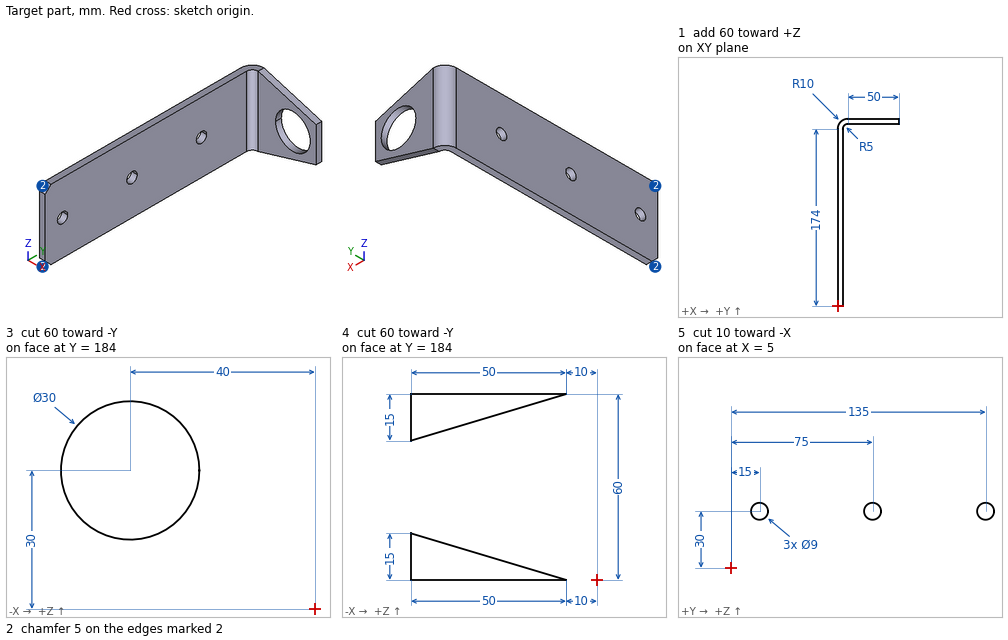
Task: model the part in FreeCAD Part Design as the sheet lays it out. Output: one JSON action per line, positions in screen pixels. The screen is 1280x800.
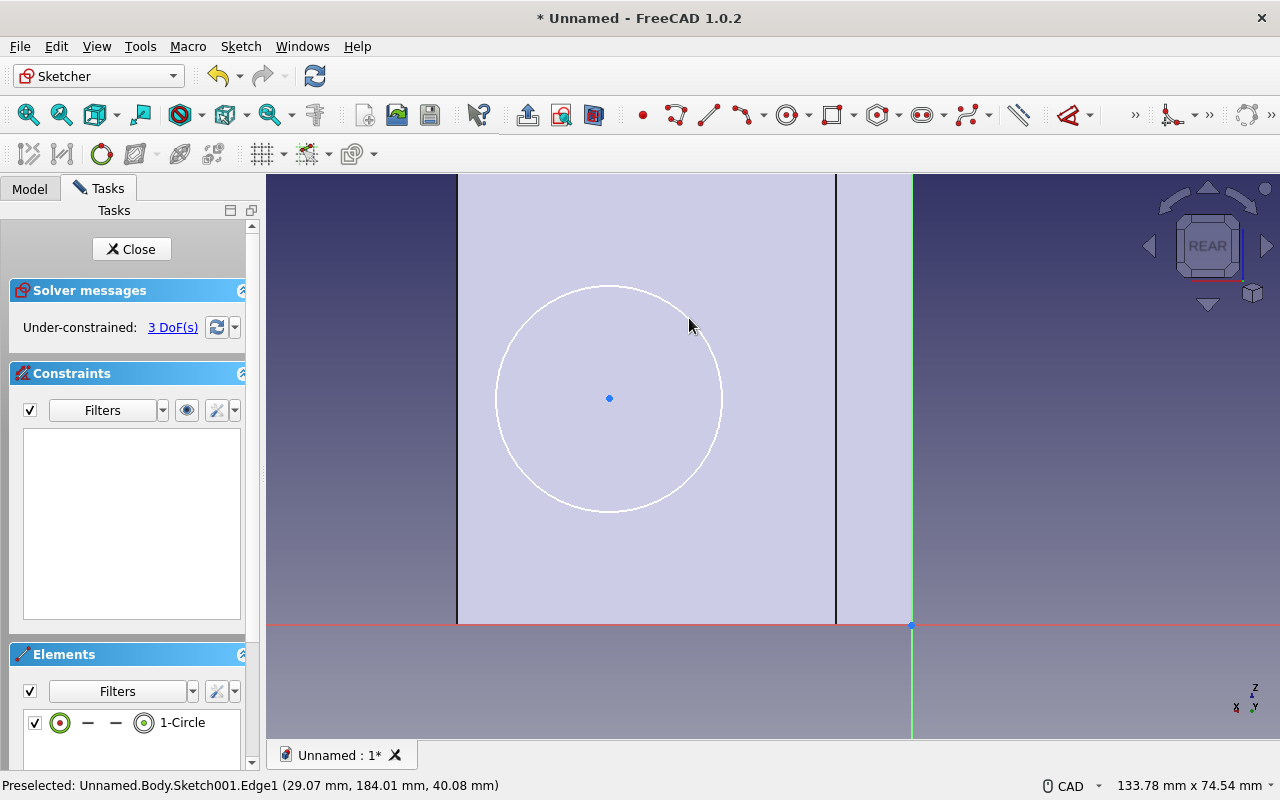
{"action": "key", "text": "d"}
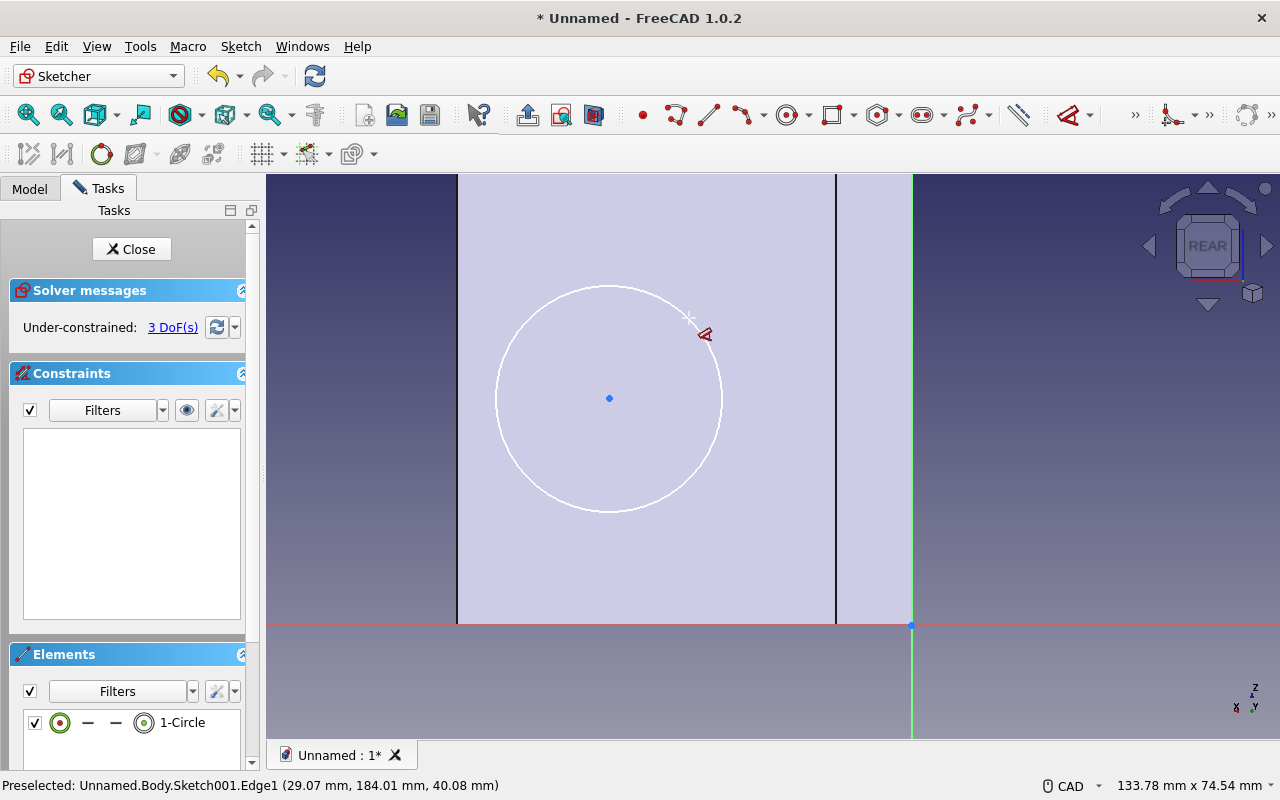
{"action": "left_click", "coordinate": [689, 319]}
{"action": "left_click", "coordinate": [712, 296]}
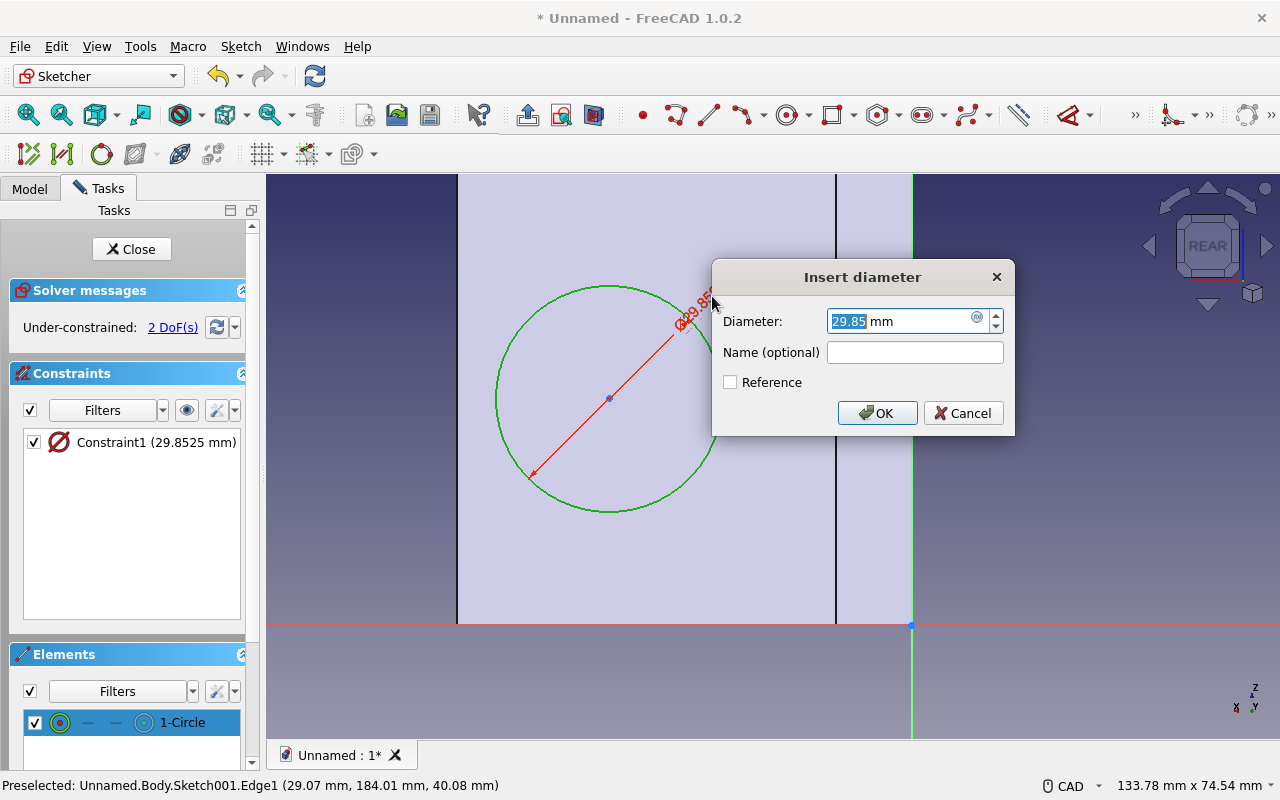
{"action": "type", "text": "30"}
{"action": "key", "text": "Return"}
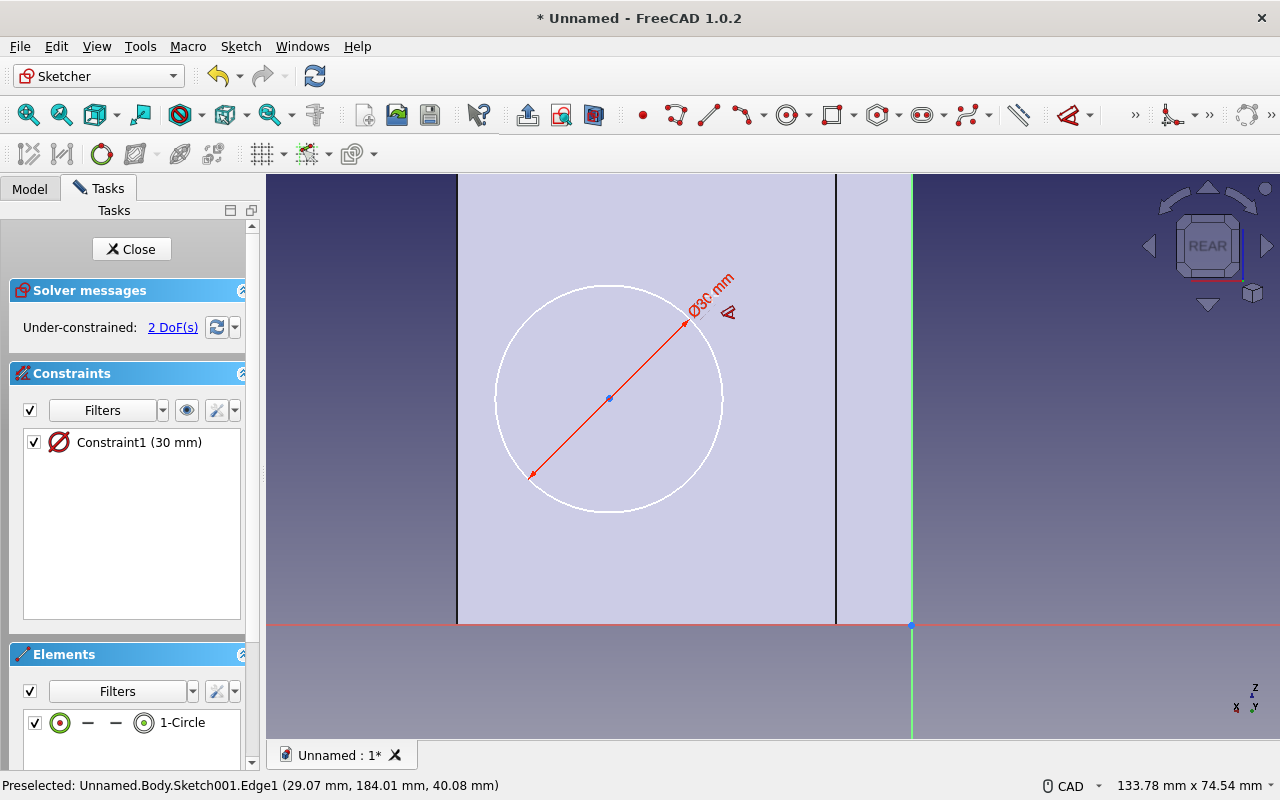
{"action": "left_click", "coordinate": [609, 399]}
{"action": "left_click", "coordinate": [760, 659]}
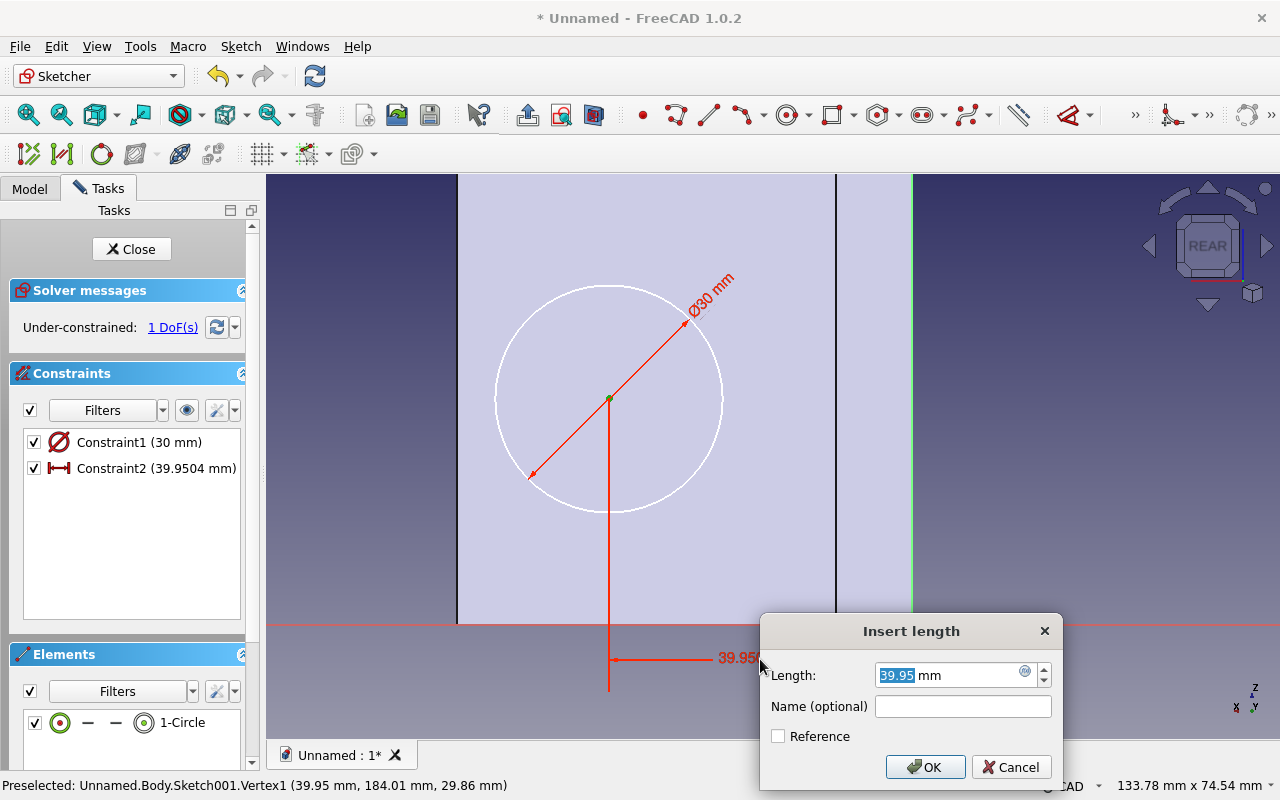
{"action": "type", "text": "40"}
{"action": "key", "text": "Return"}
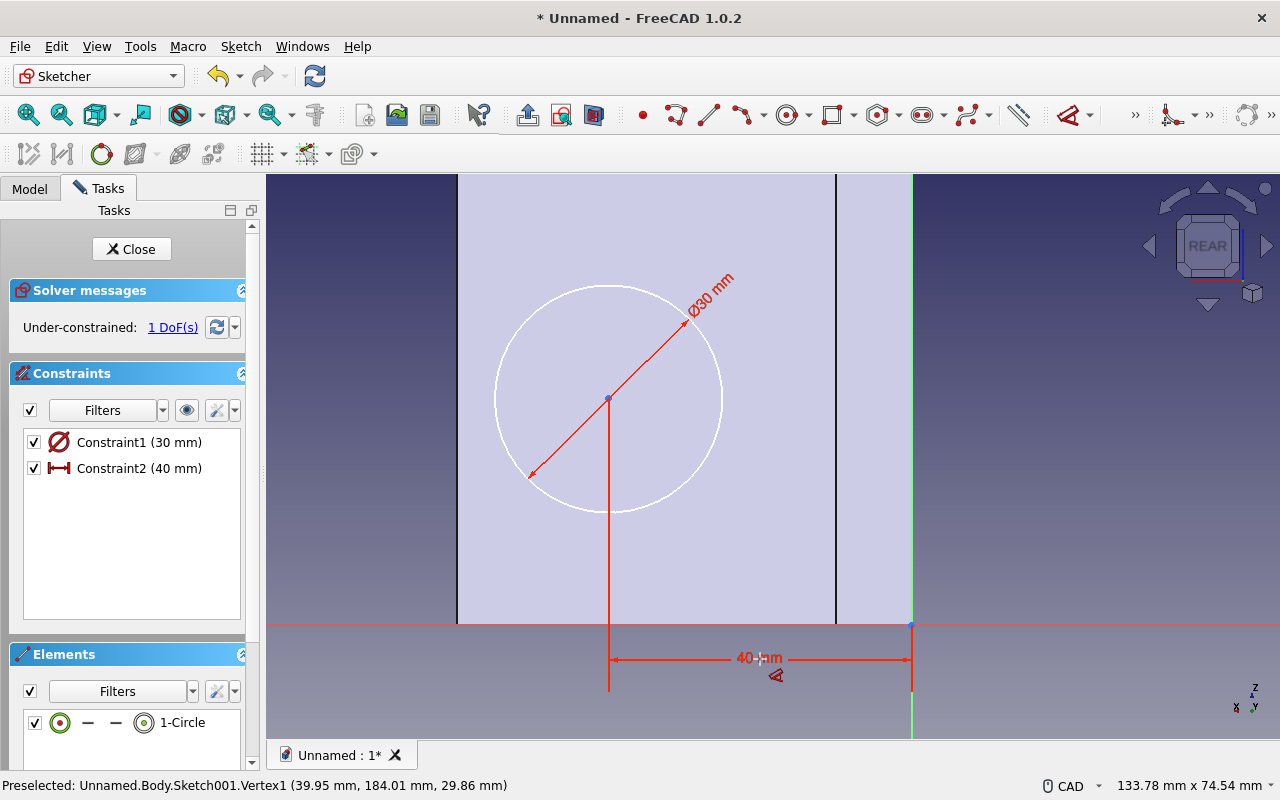
{"action": "left_click", "coordinate": [609, 399]}
{"action": "left_click", "coordinate": [946, 512]}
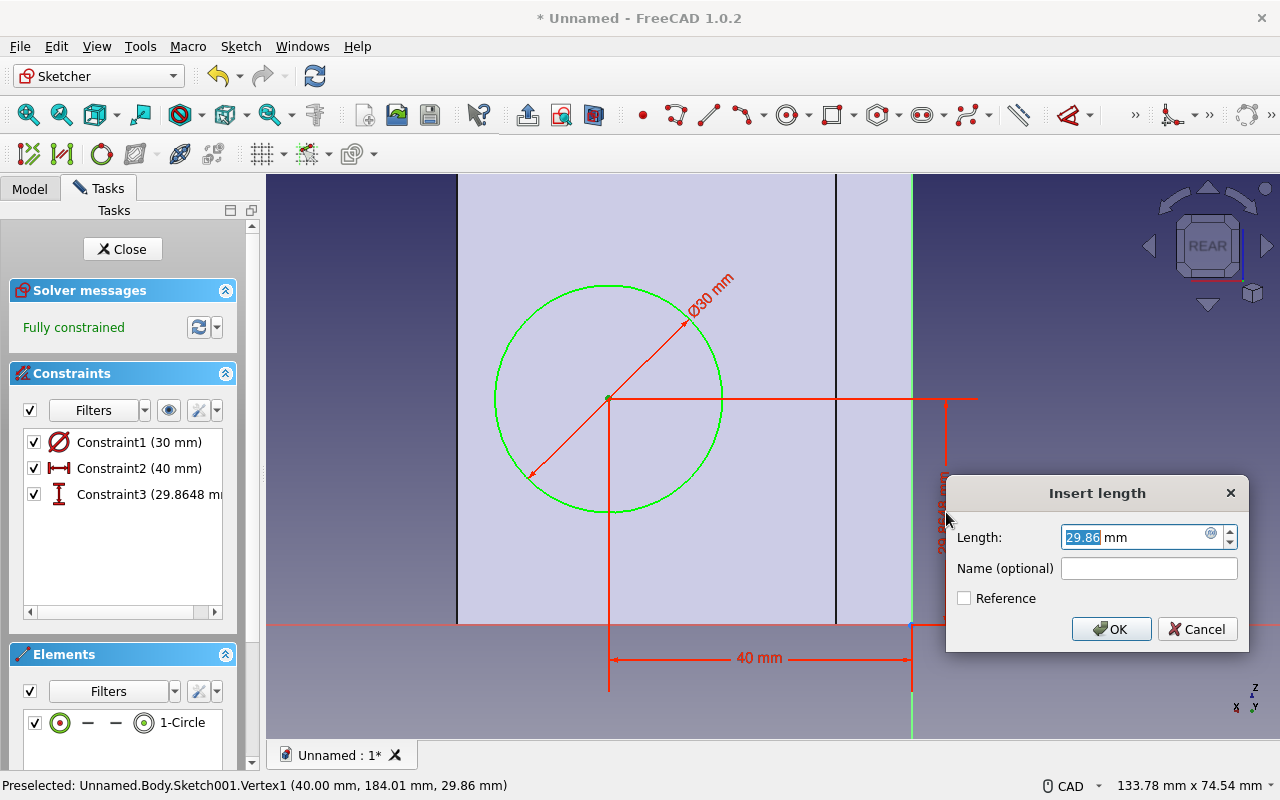
{"action": "type", "text": "30"}
{"action": "key", "text": "Return"}
{"action": "key", "text": "Escape"}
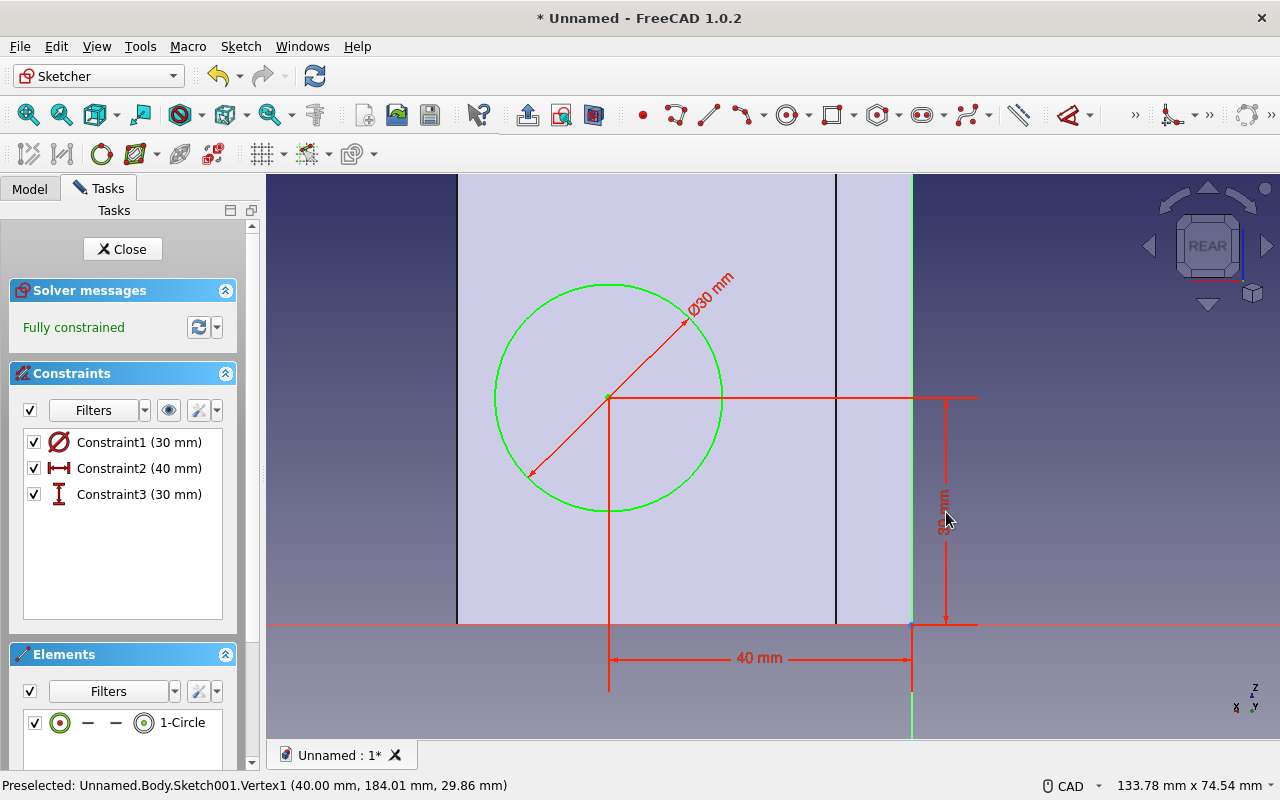
{"action": "left_click", "coordinate": [123, 249]}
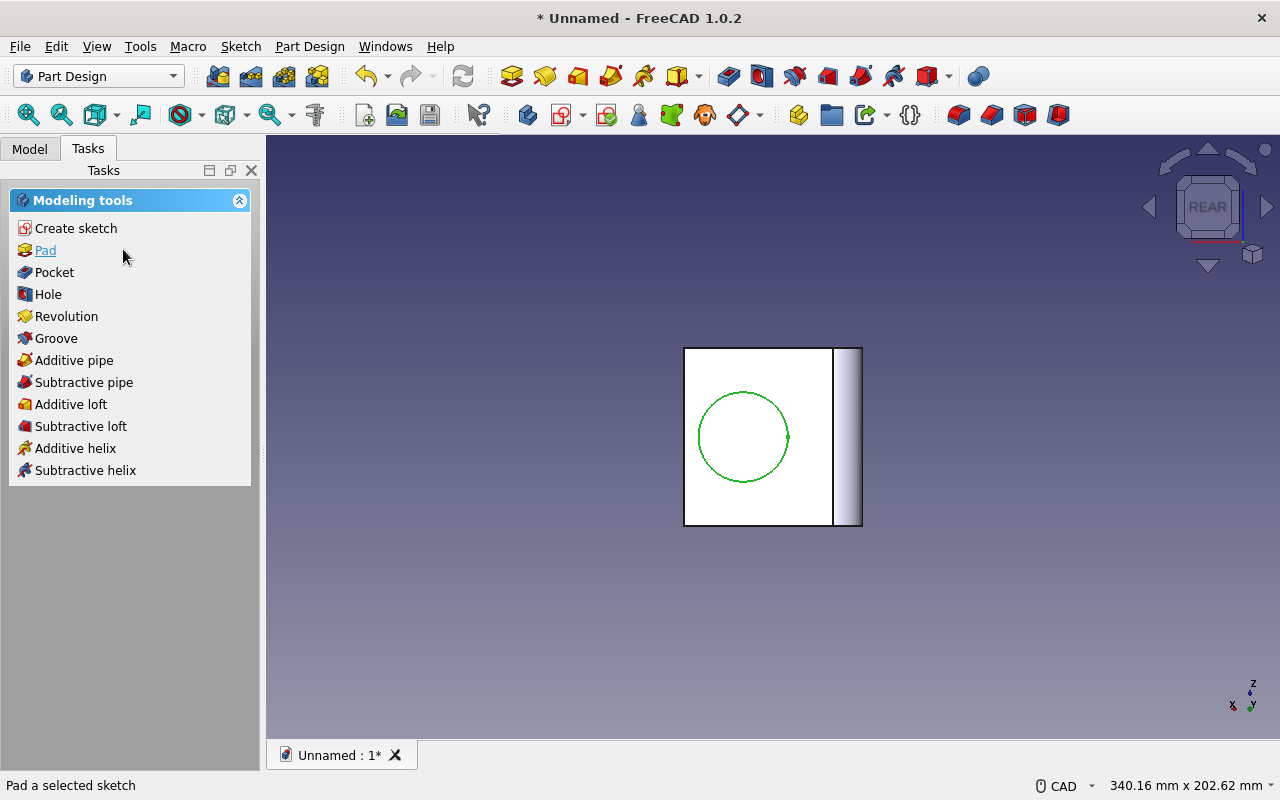
{"action": "left_click", "coordinate": [729, 76]}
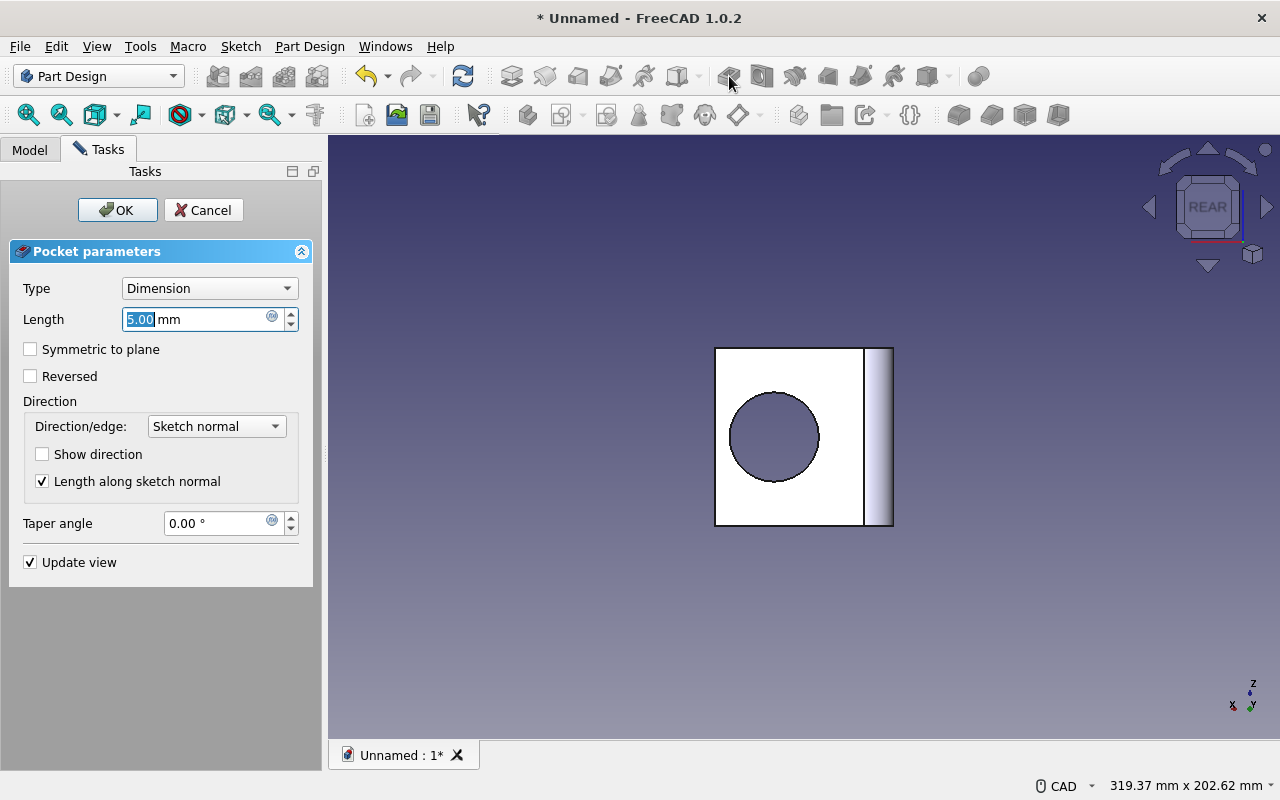
{"action": "type", "text": "60"}
{"action": "key", "text": "Tab"}